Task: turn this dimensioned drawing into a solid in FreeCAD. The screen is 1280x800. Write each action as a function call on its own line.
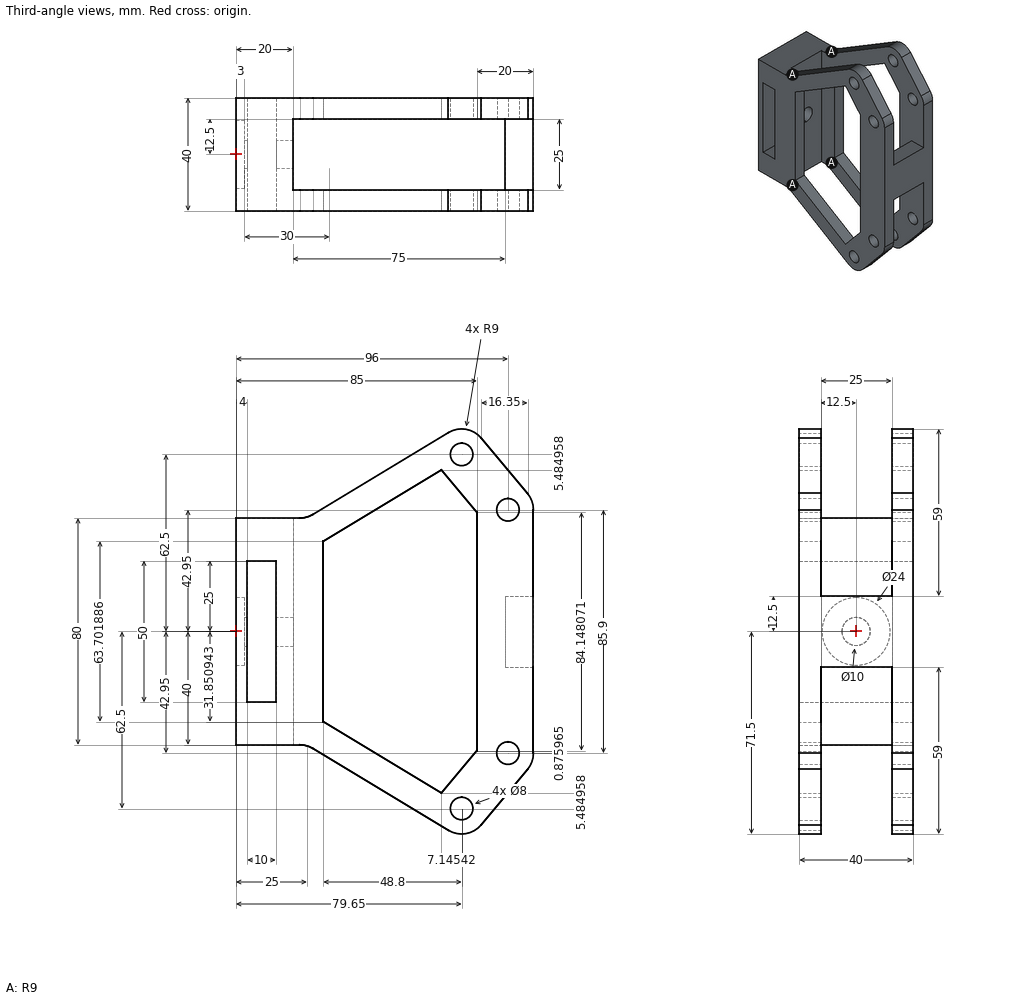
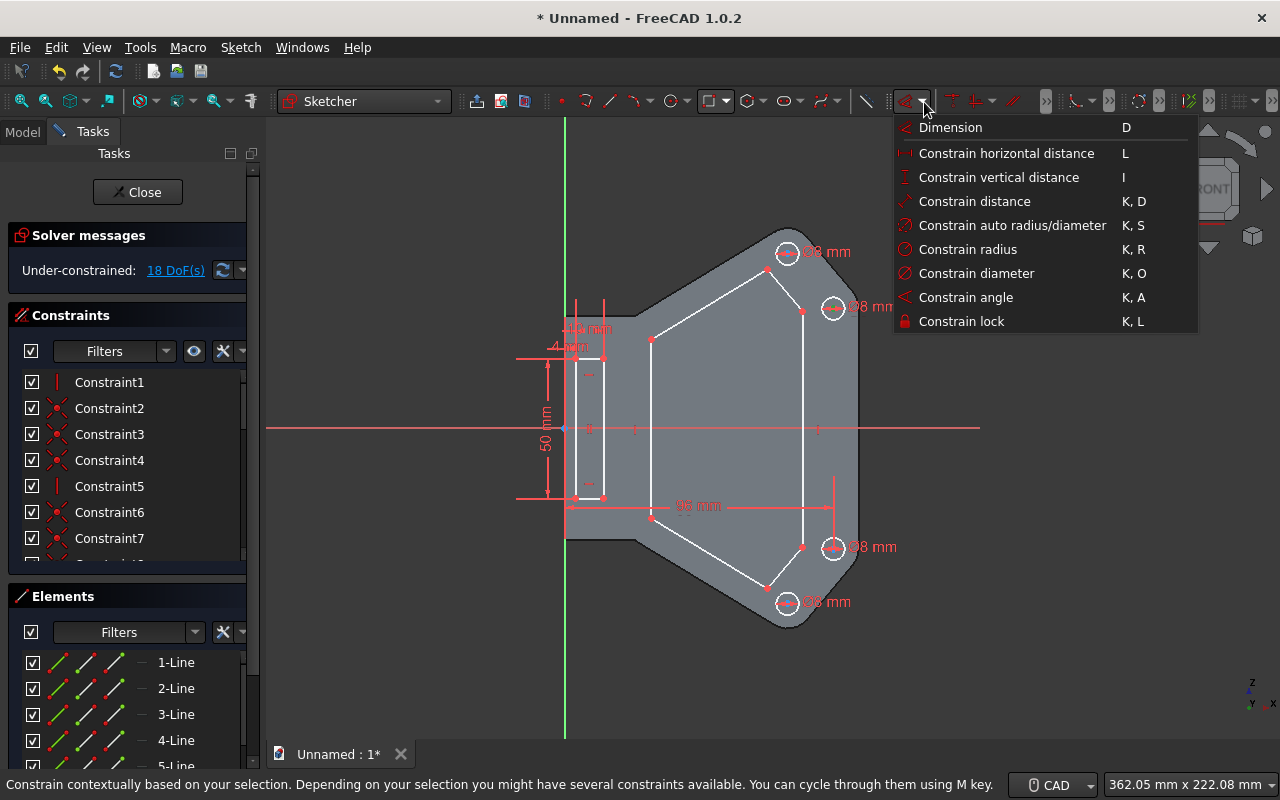
click(1046, 153)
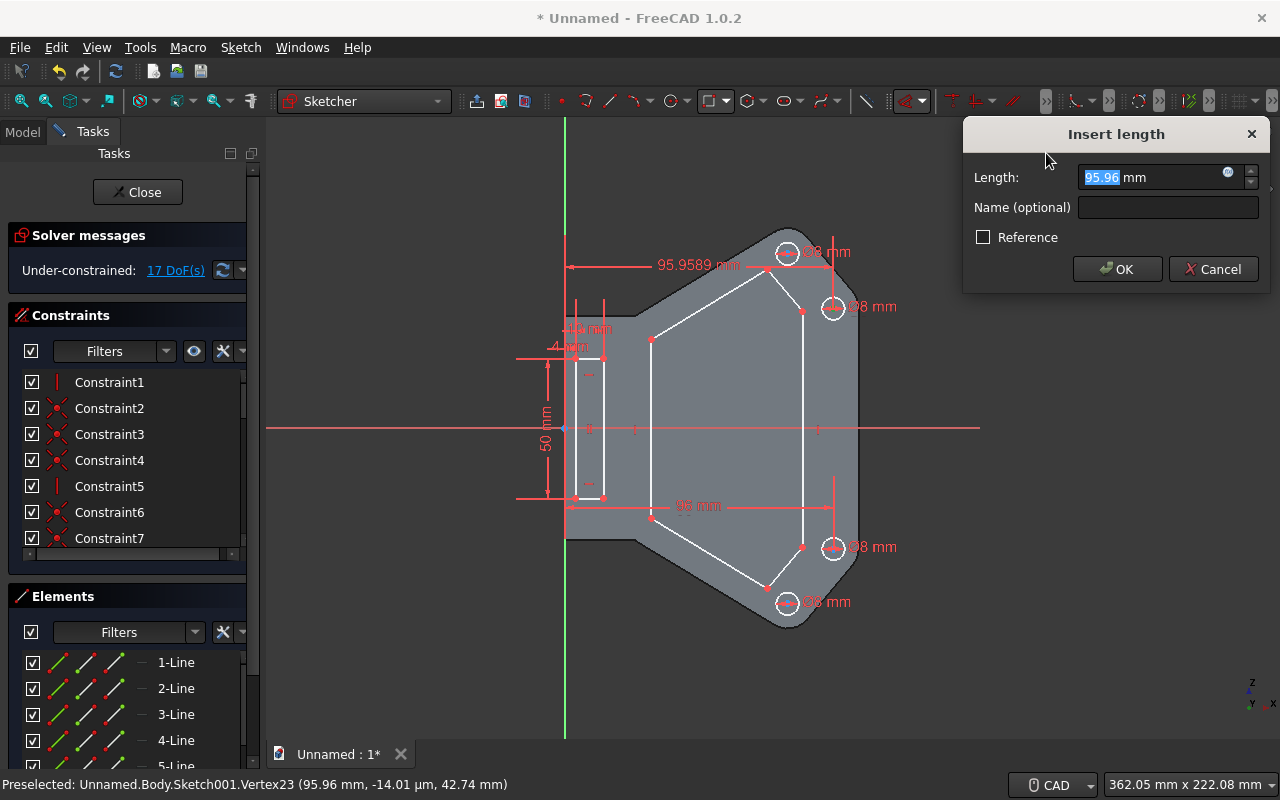
text(96)
key(Return)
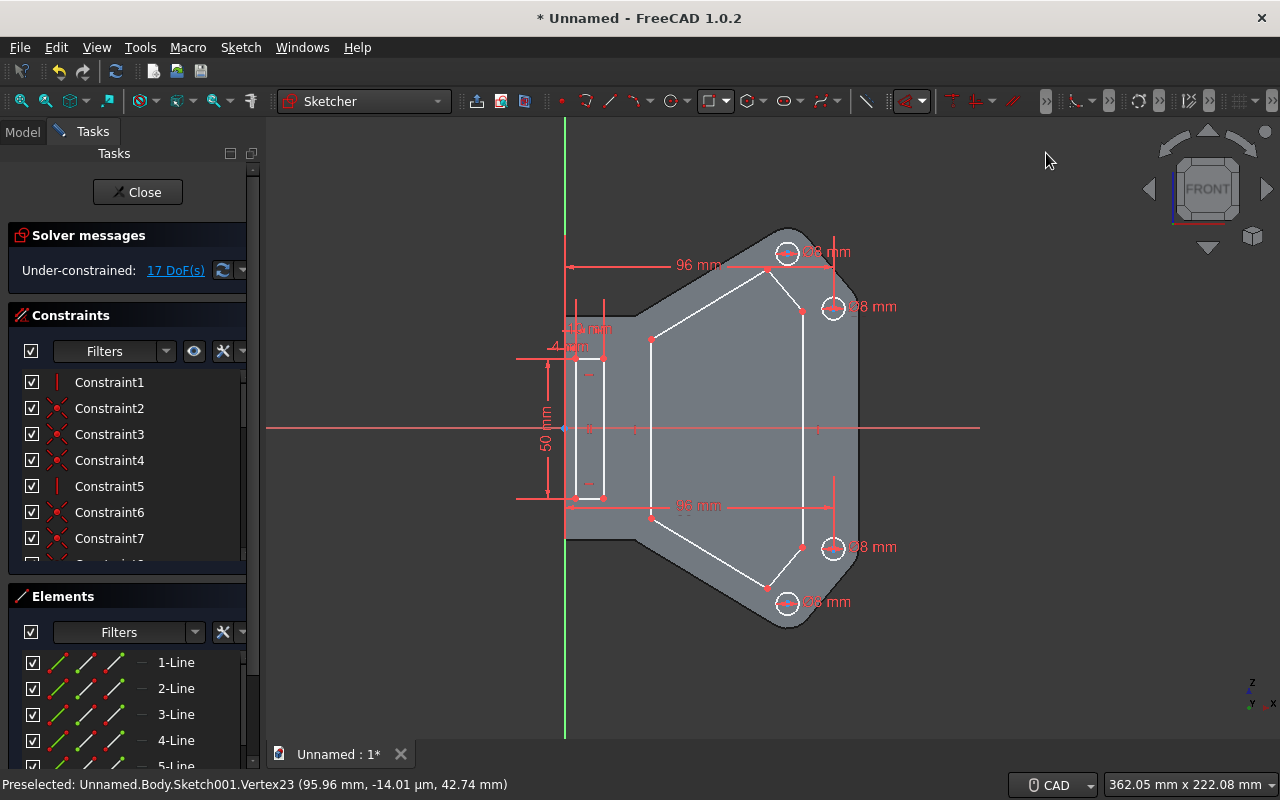
click(803, 311)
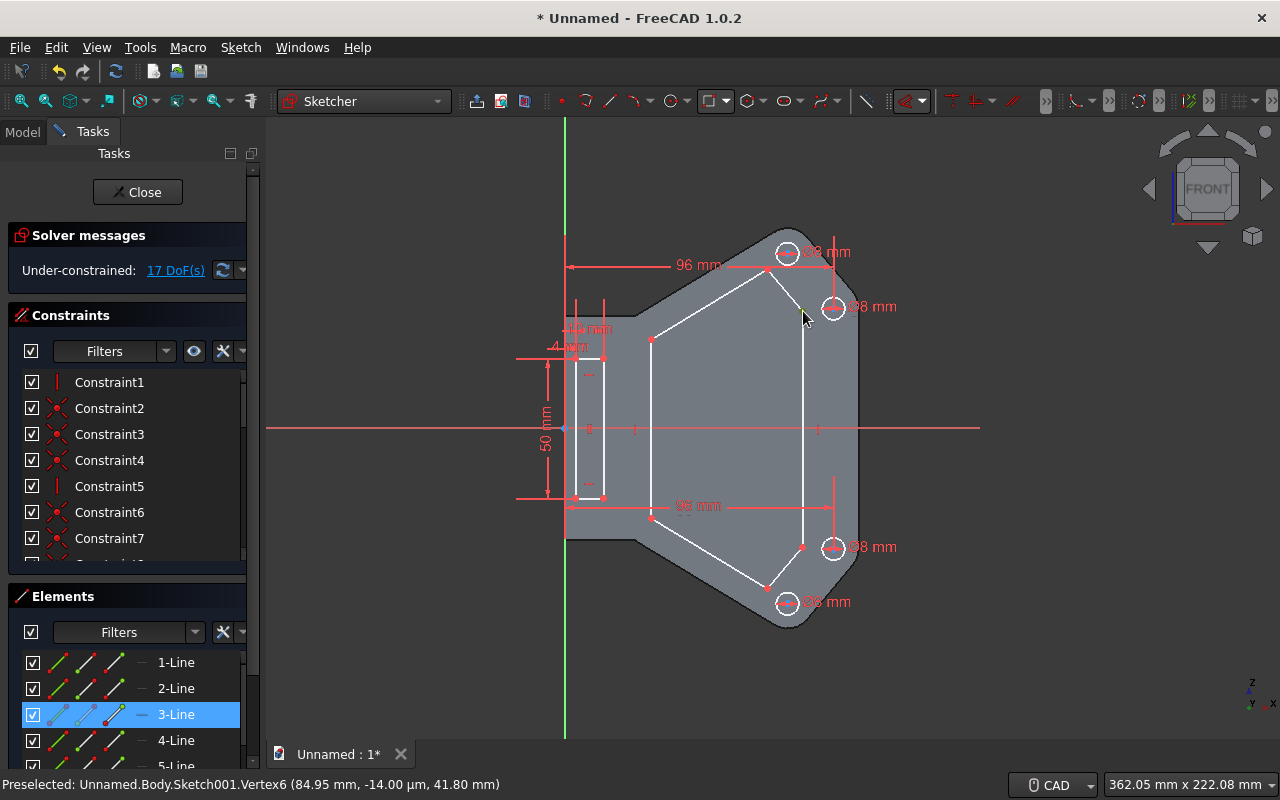
key(l)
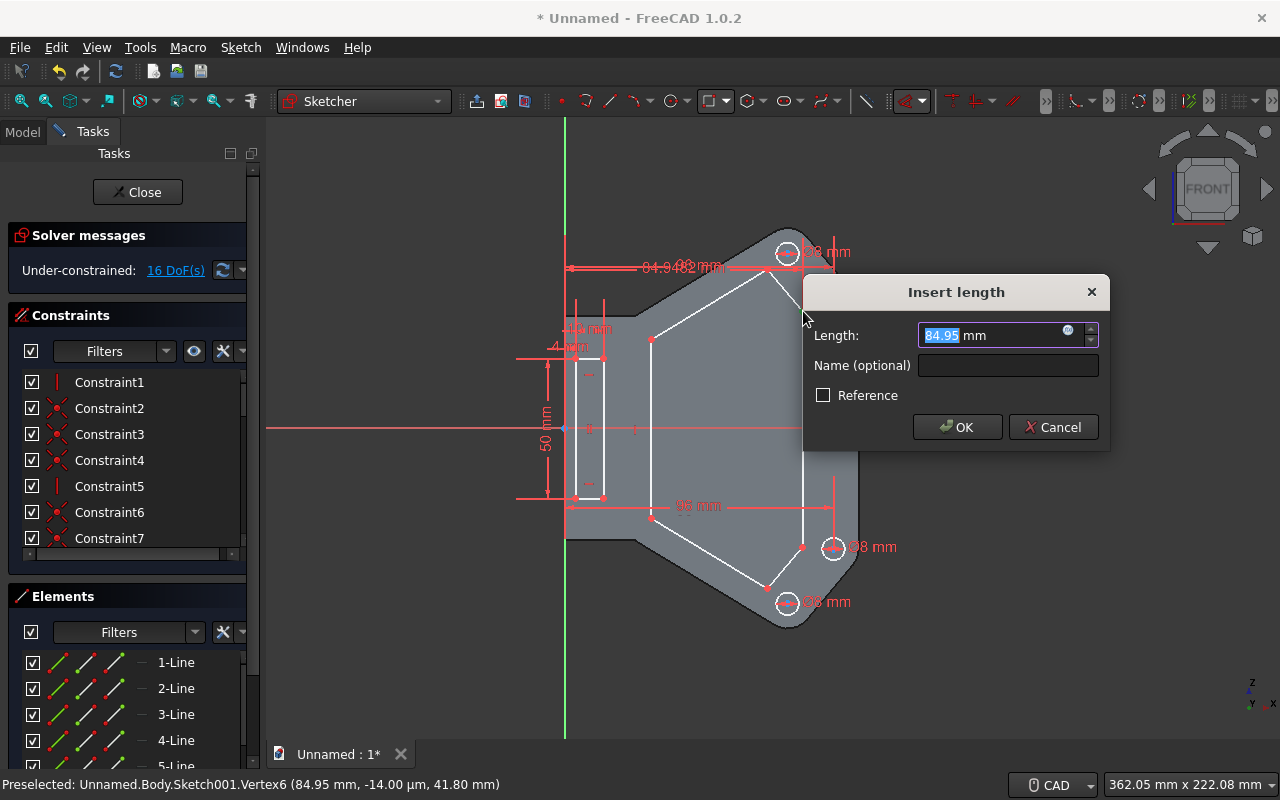
text(85)
key(Return)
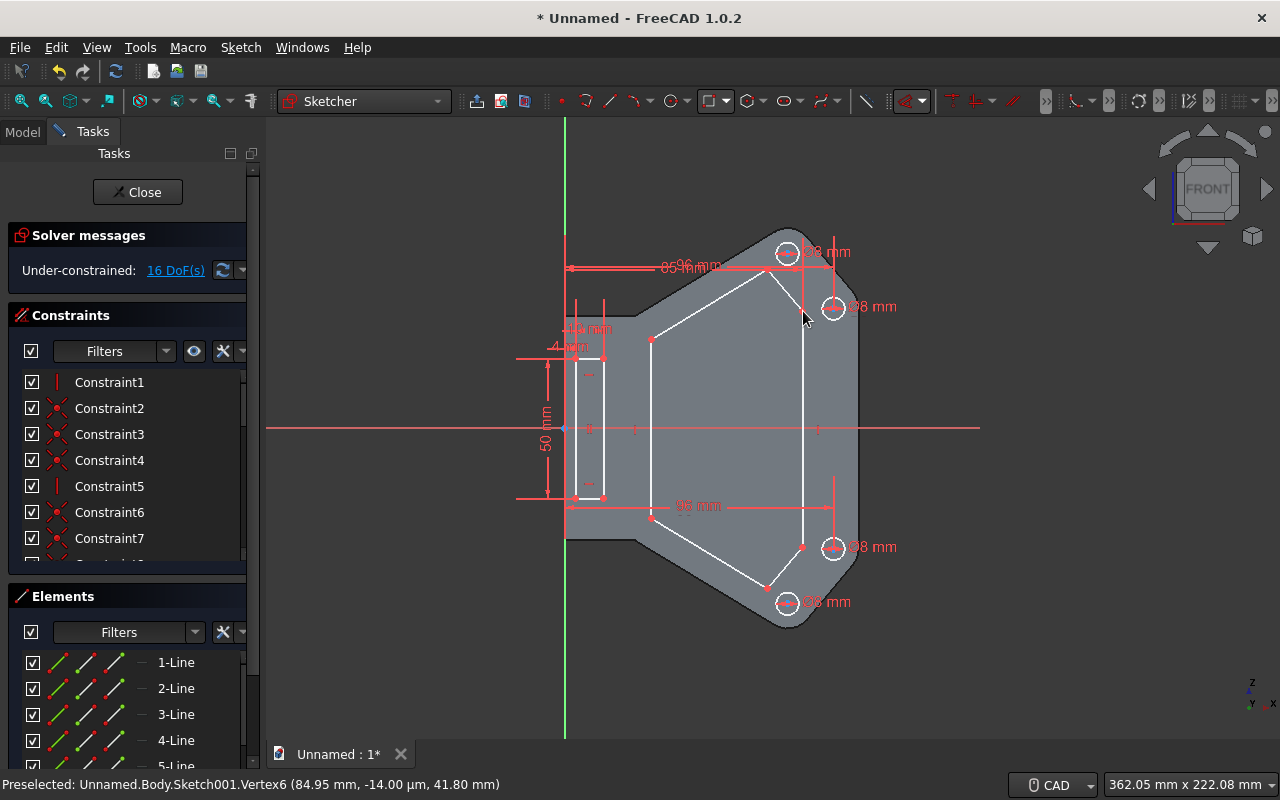
click(576, 359)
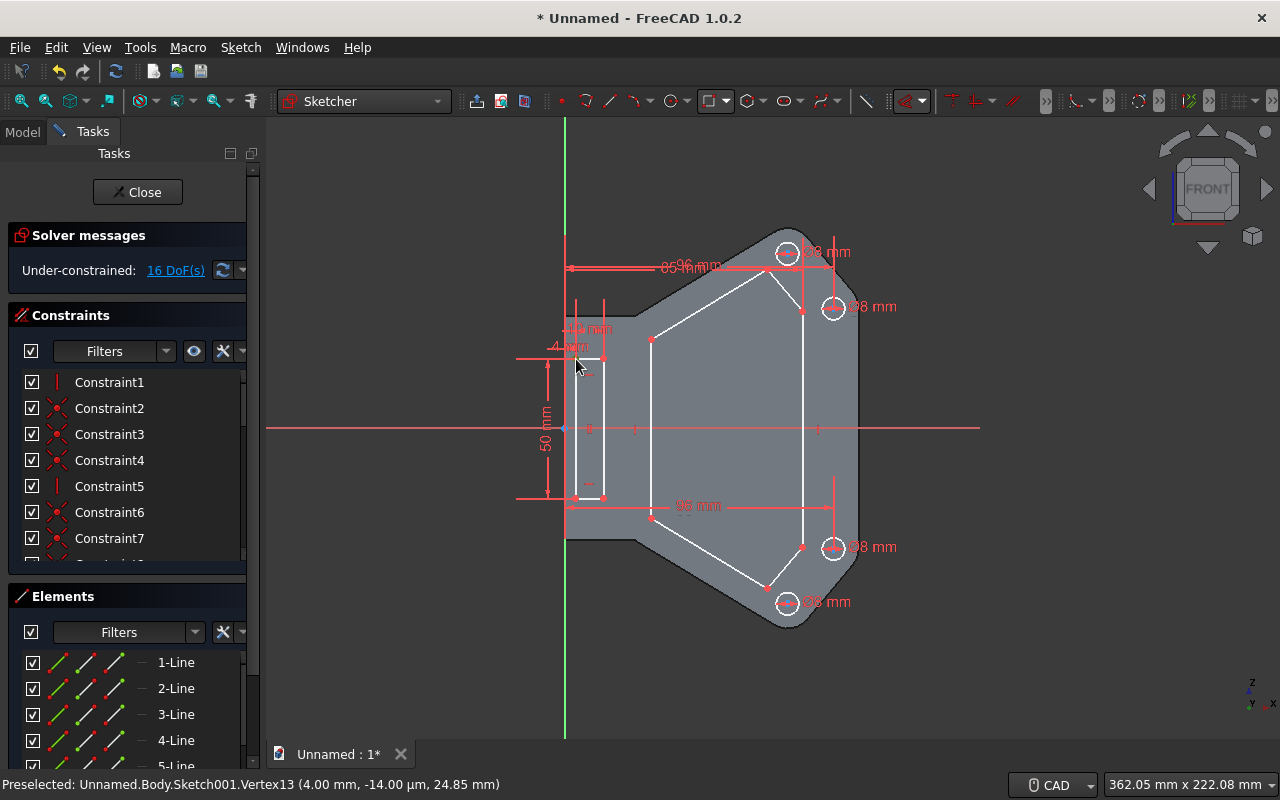
key(i)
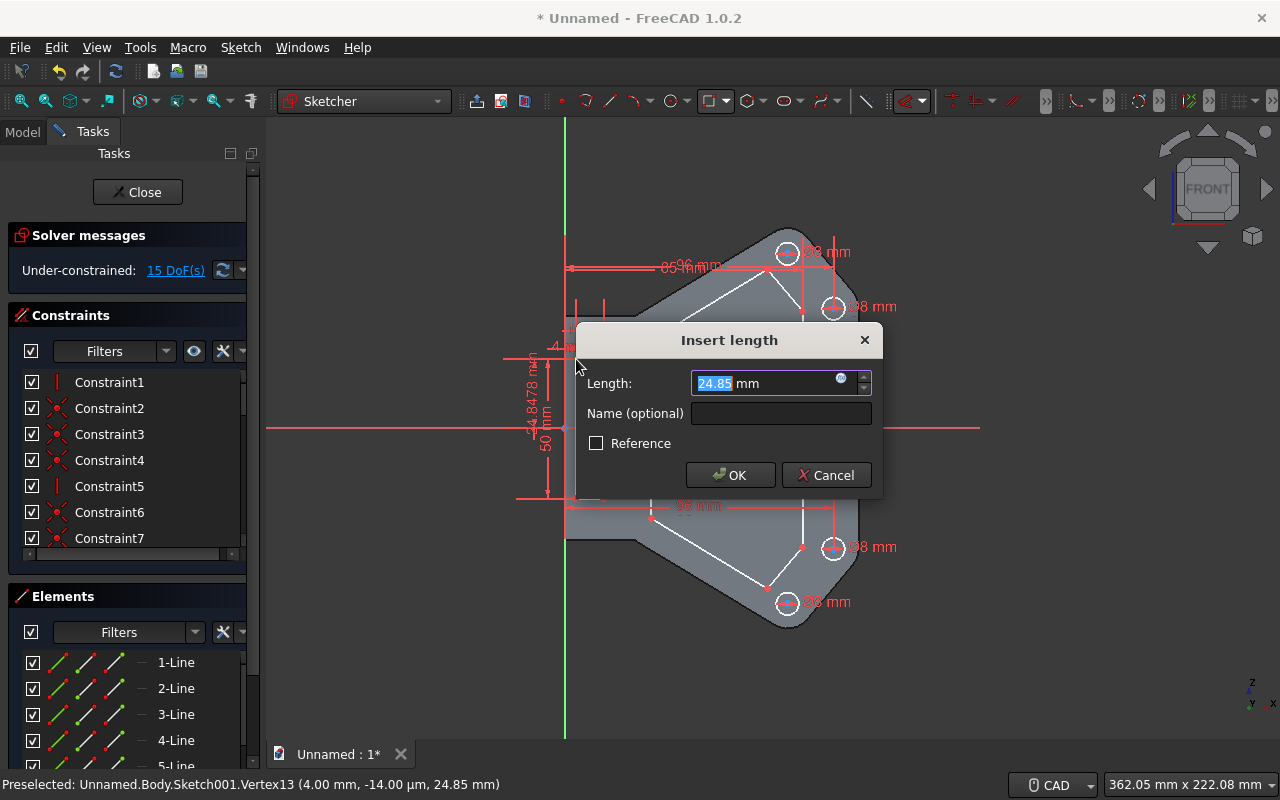
text(25)
key(Return)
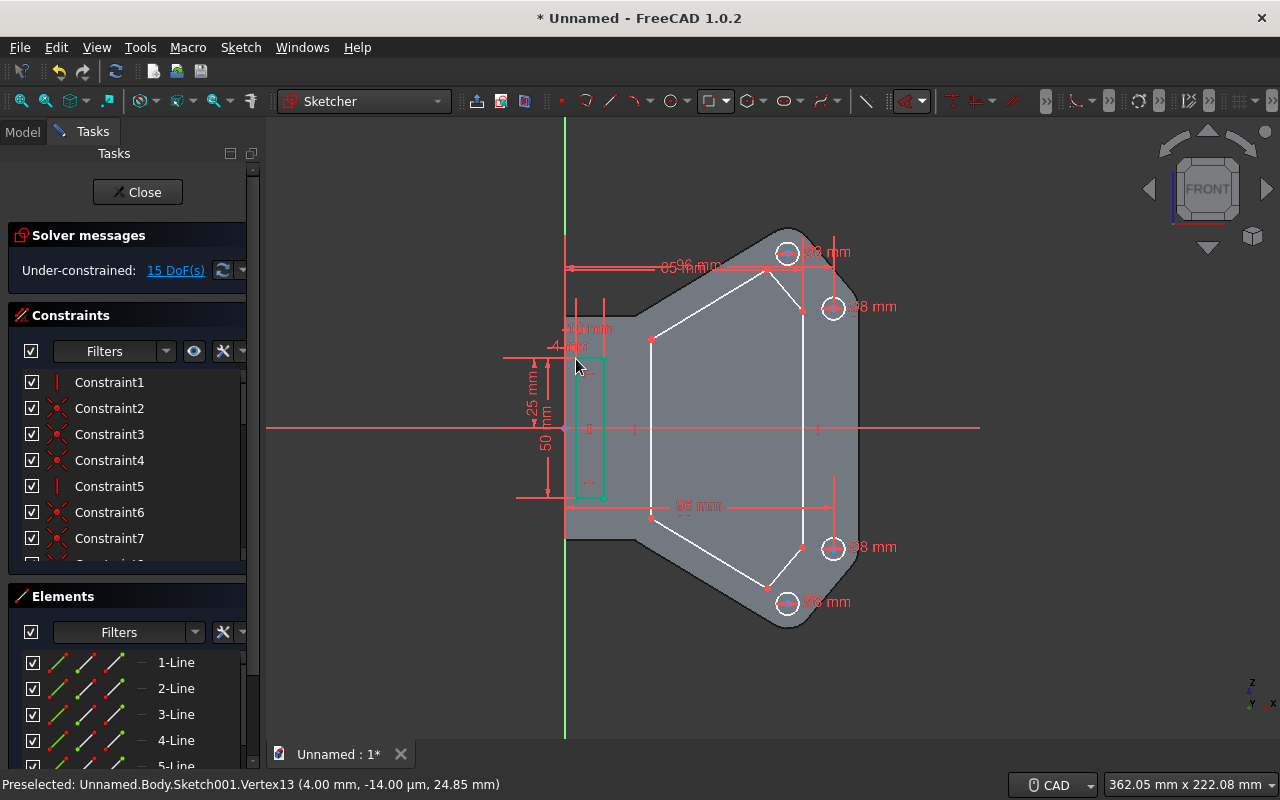
click(788, 604)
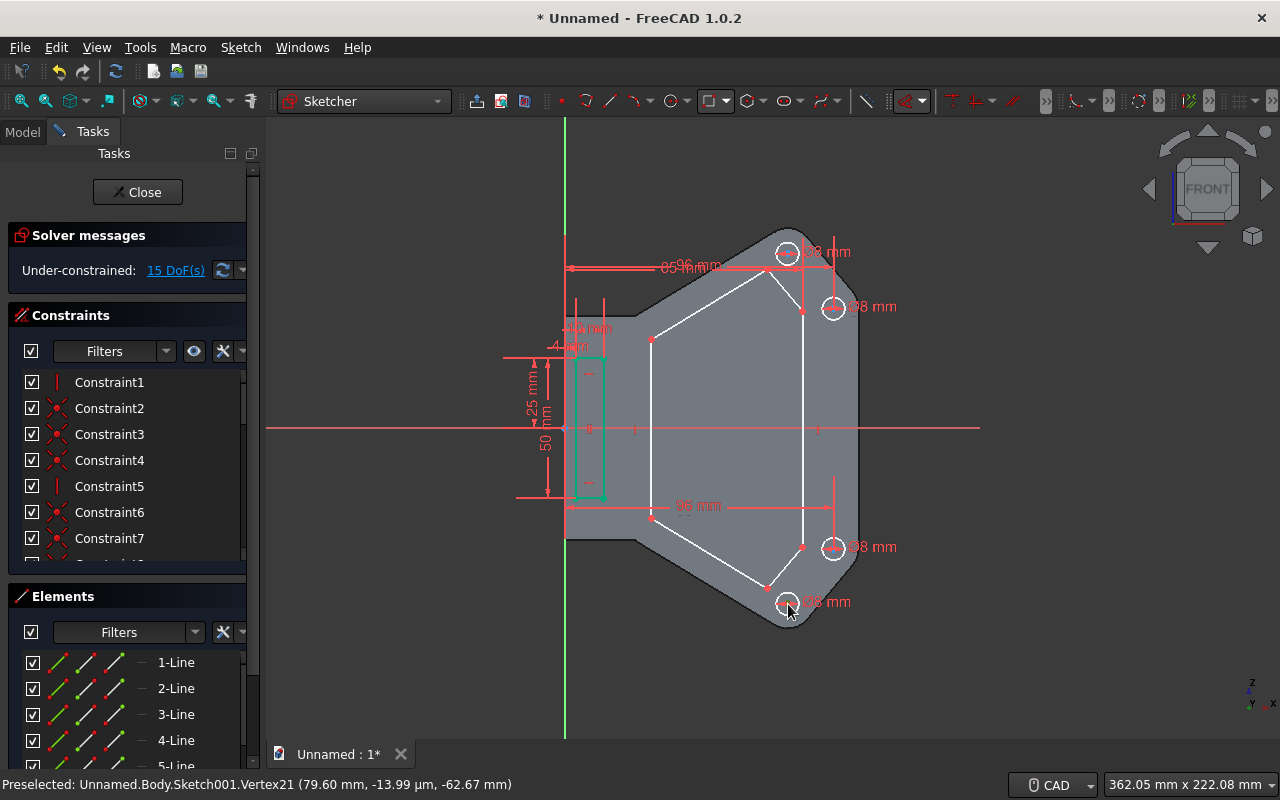
click(924, 102)